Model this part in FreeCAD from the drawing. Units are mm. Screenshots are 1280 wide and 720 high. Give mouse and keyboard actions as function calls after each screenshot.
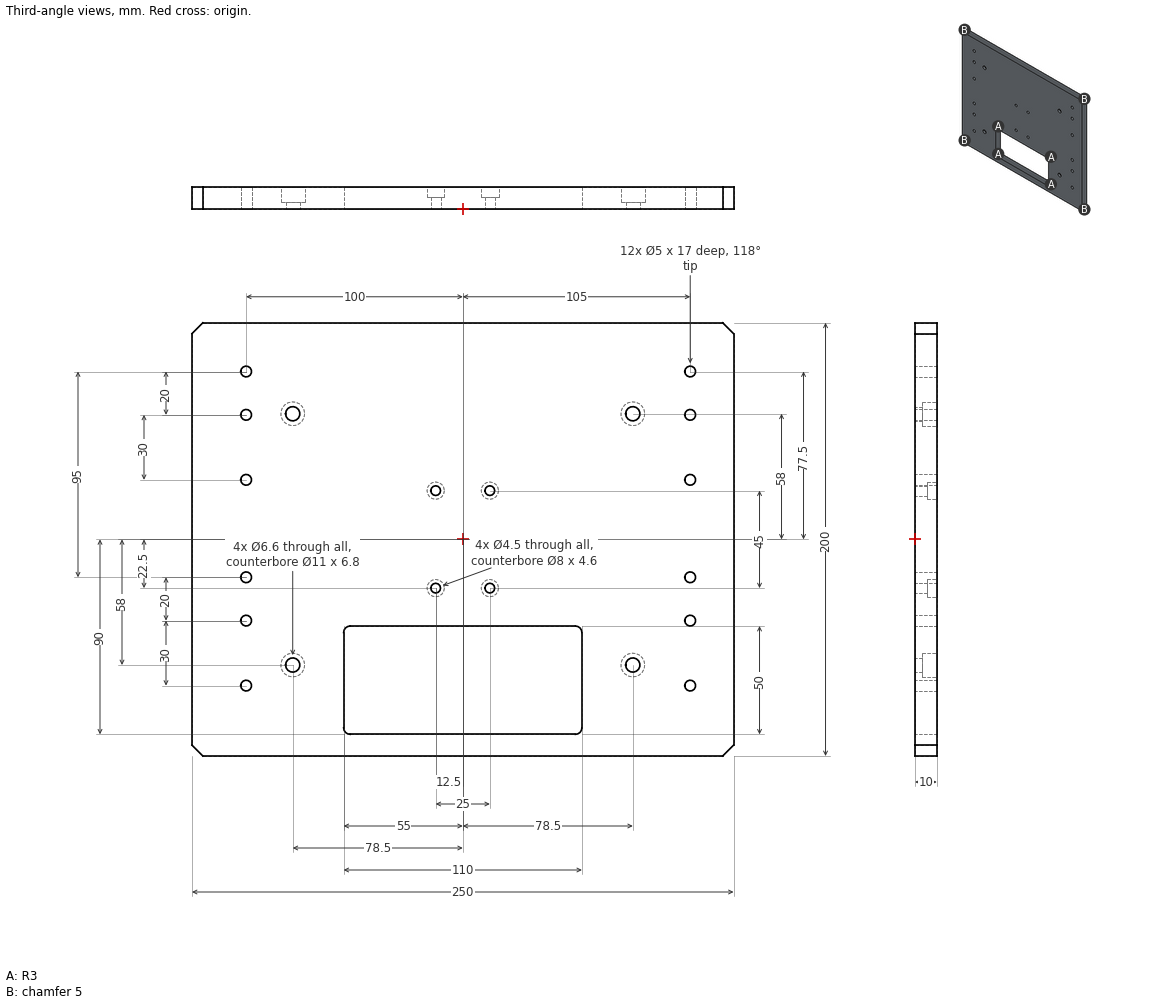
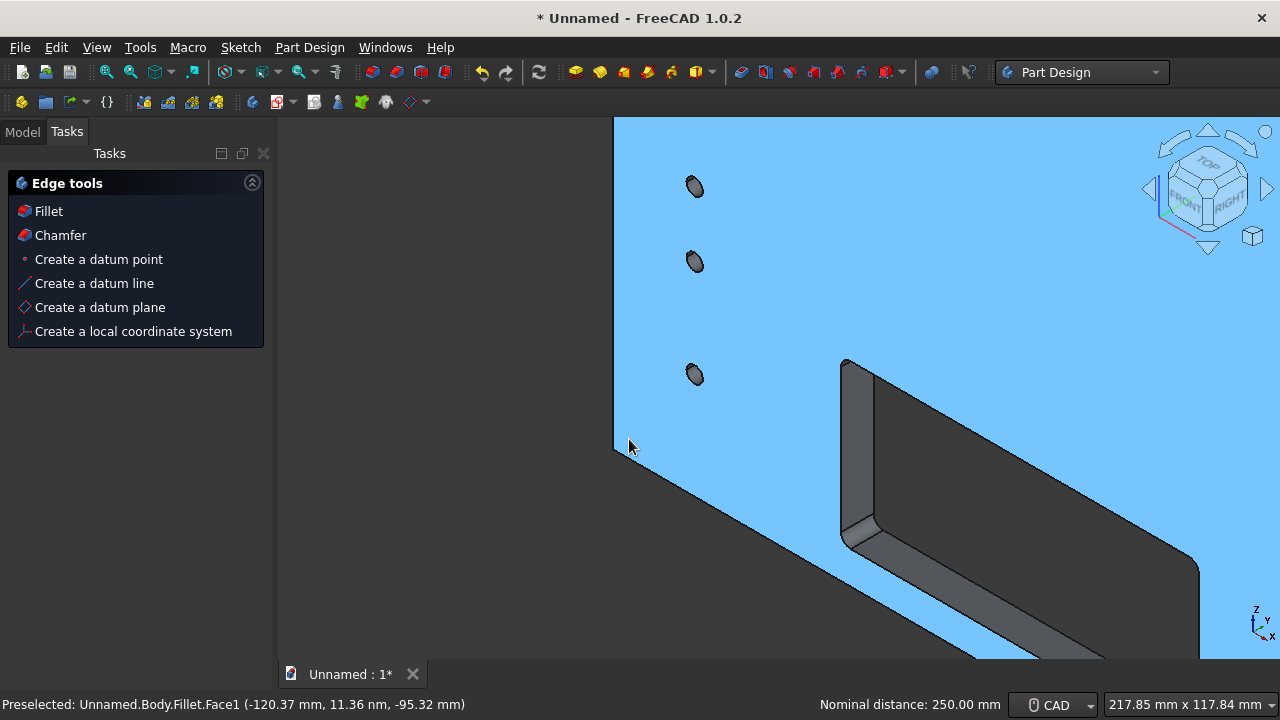
click(108, 72)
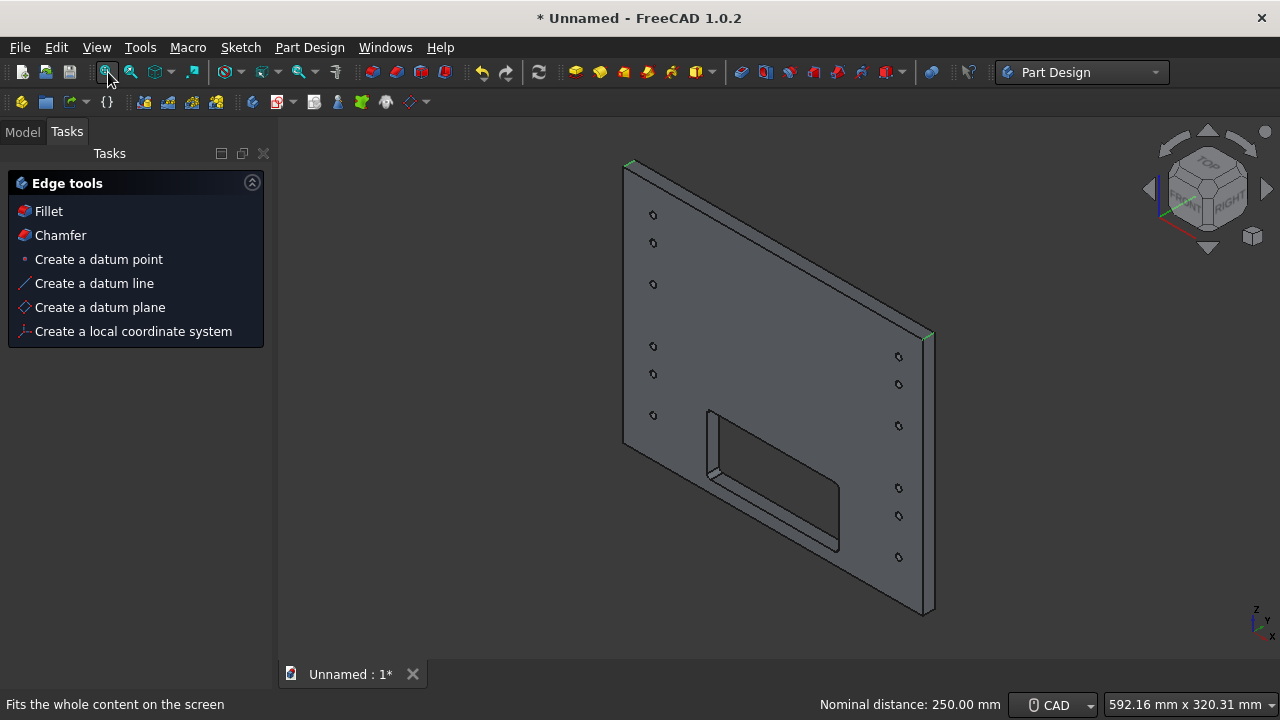
key(1)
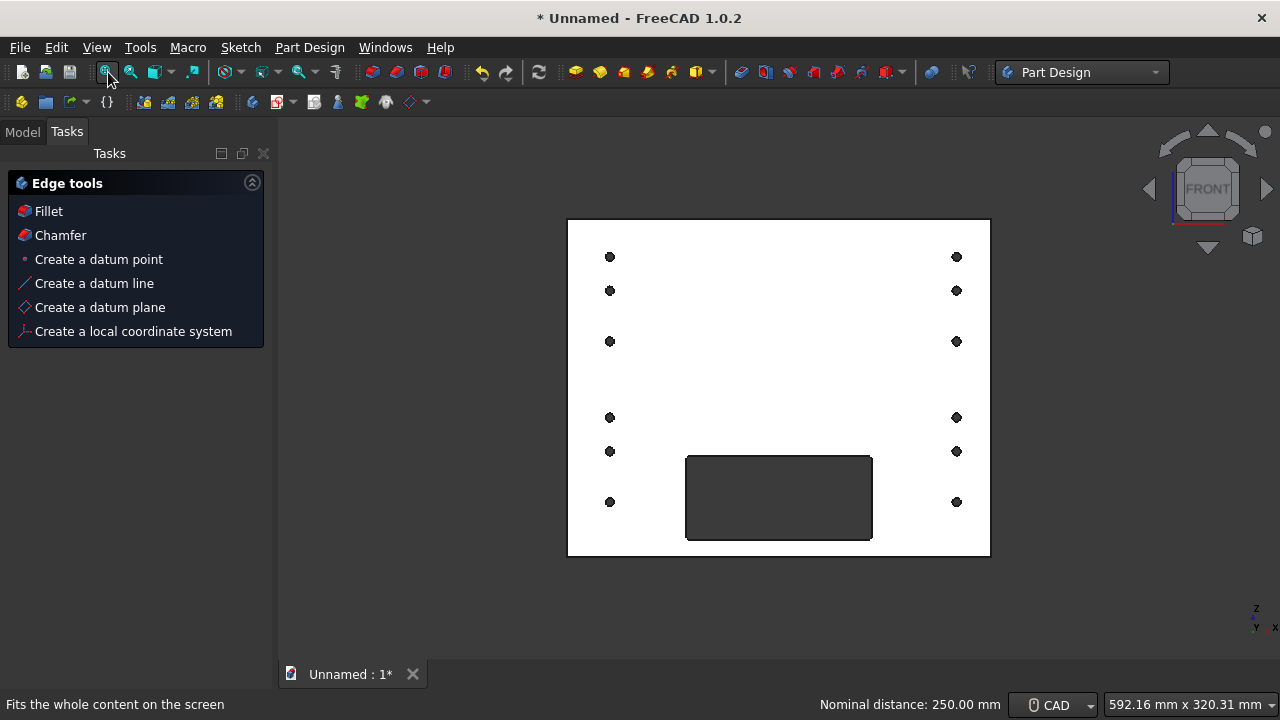
scroll(567, 556, up, 5)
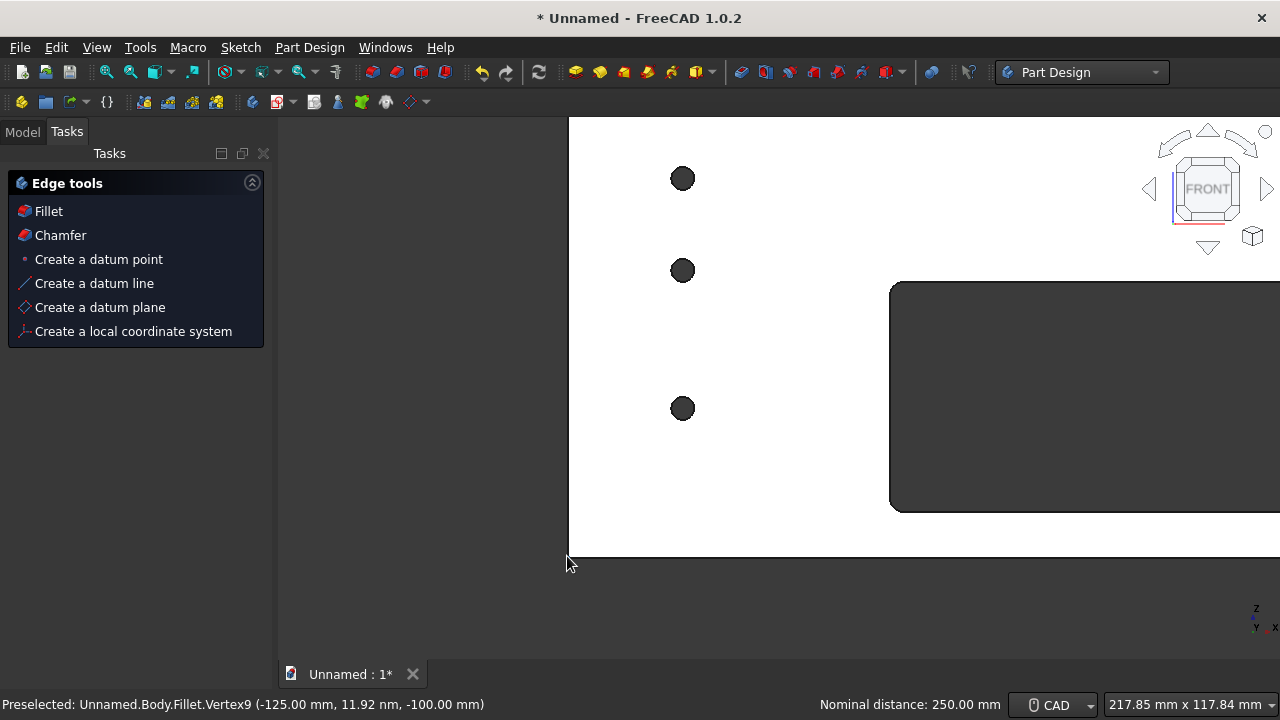
click(108, 72)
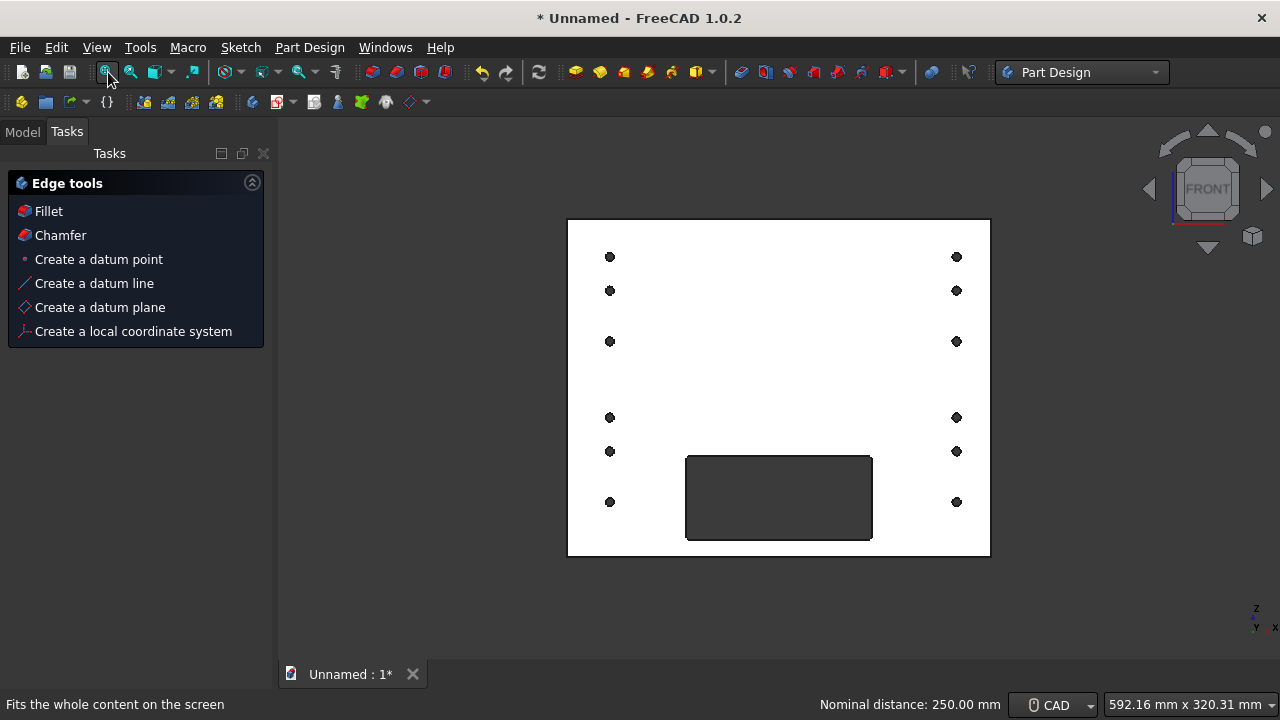
key(3)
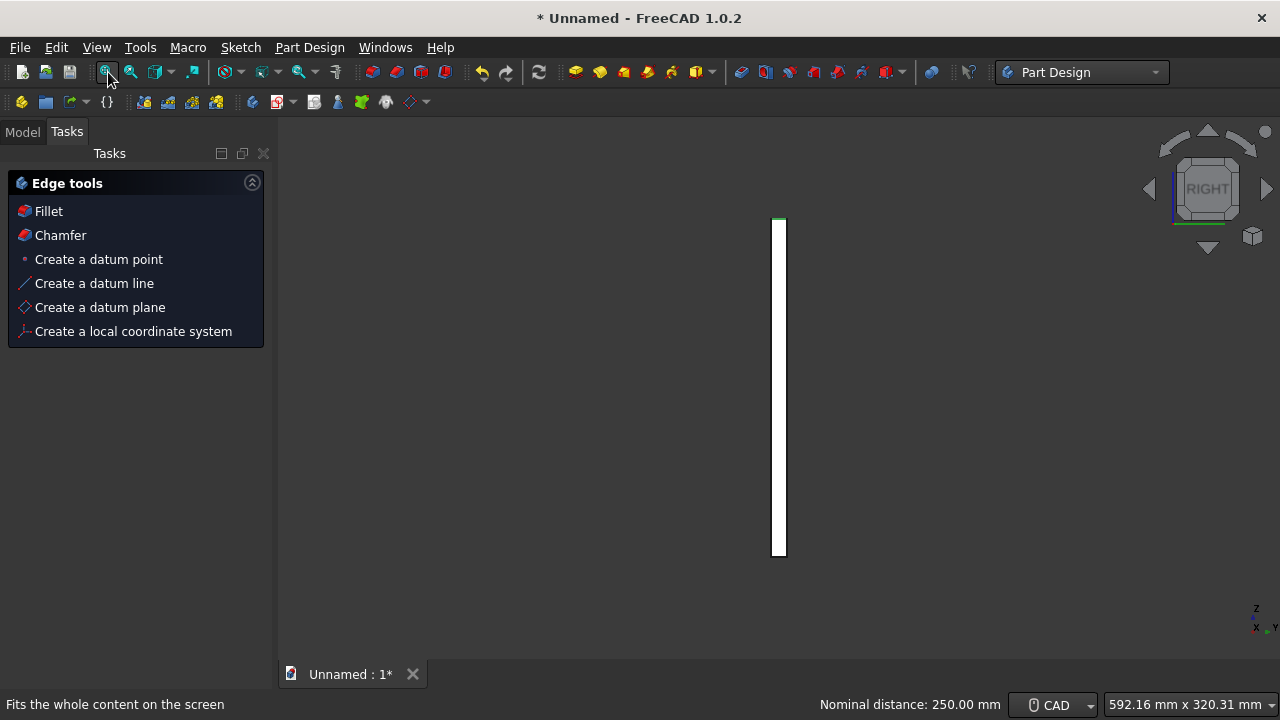
click(779, 556, ctrl)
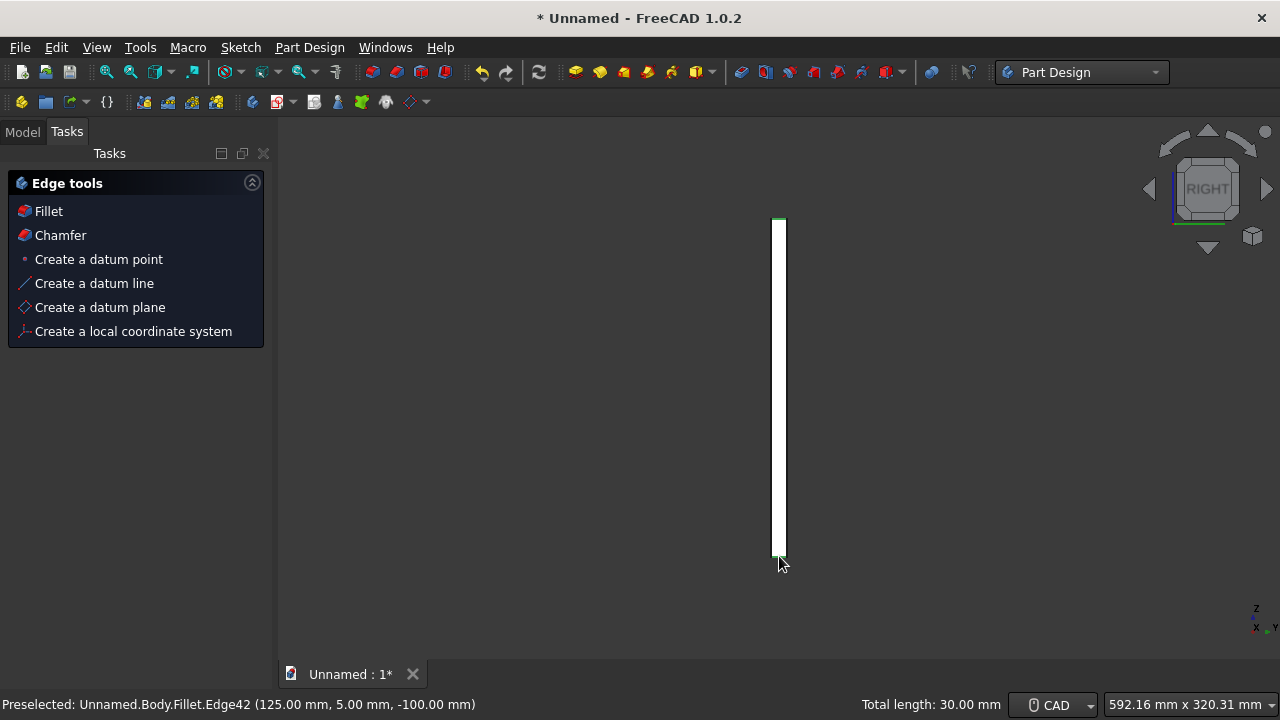
scroll(779, 556, up, 5)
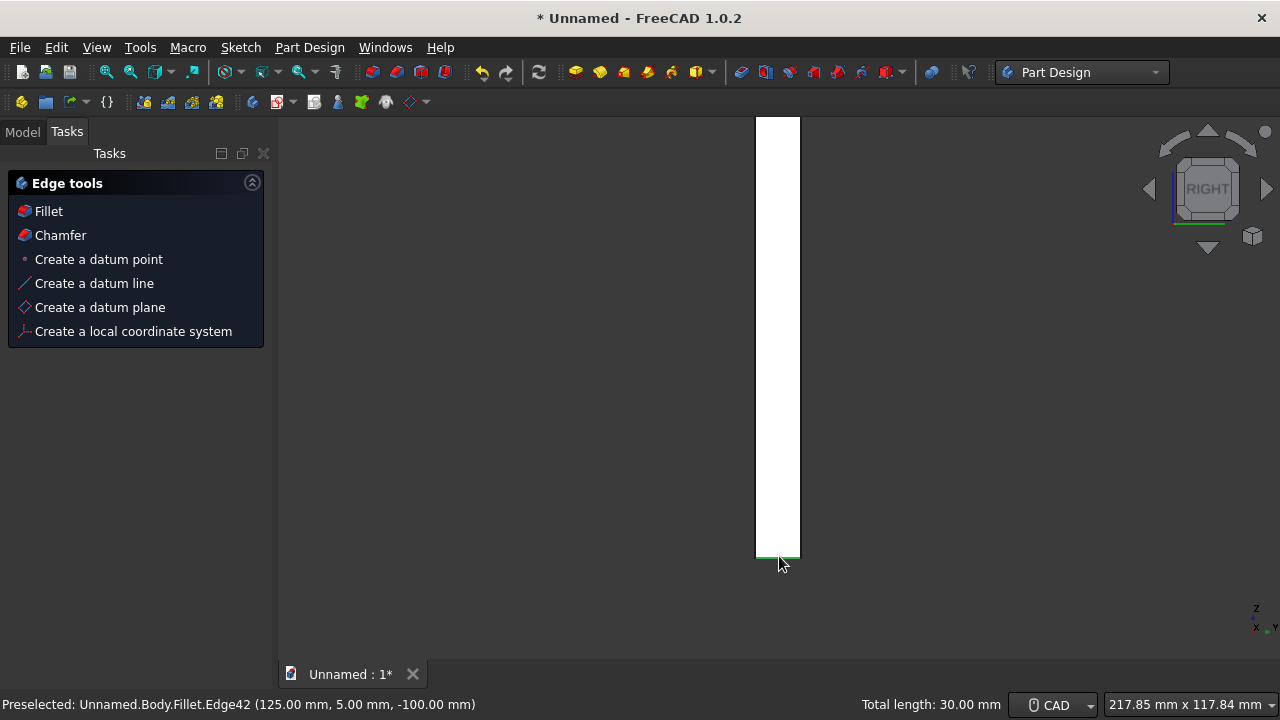
click(108, 72)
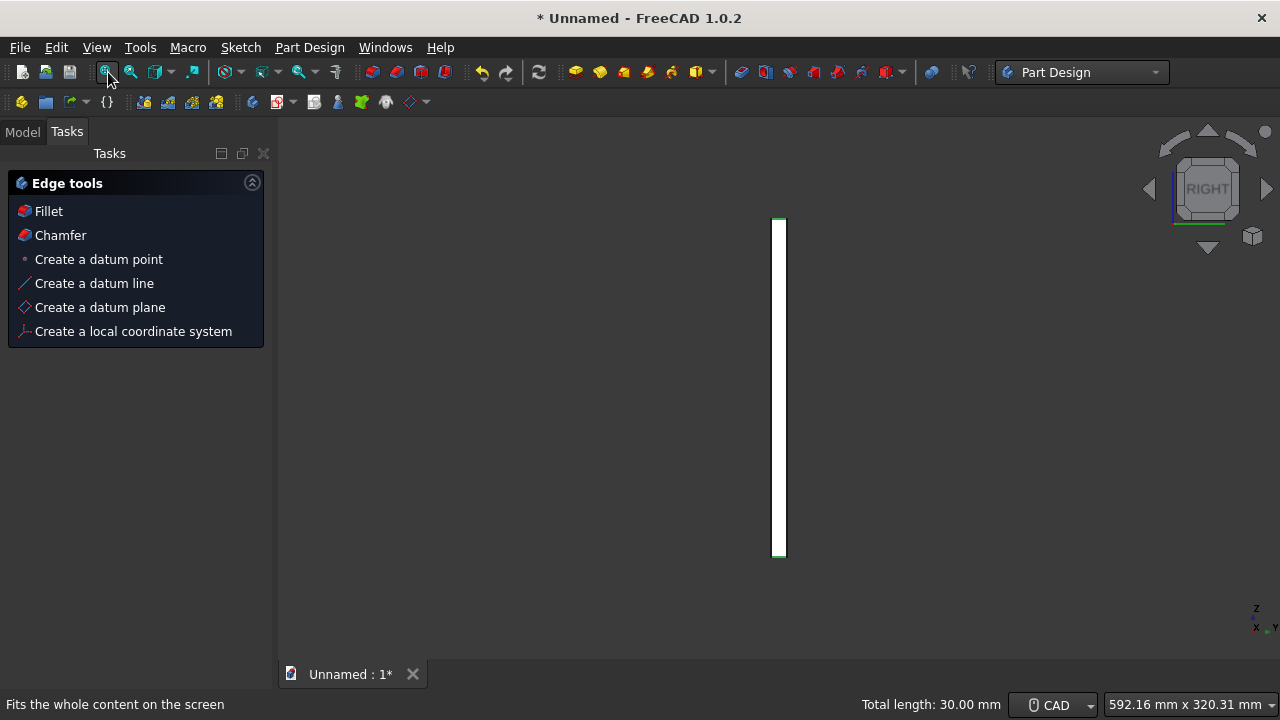
key(5)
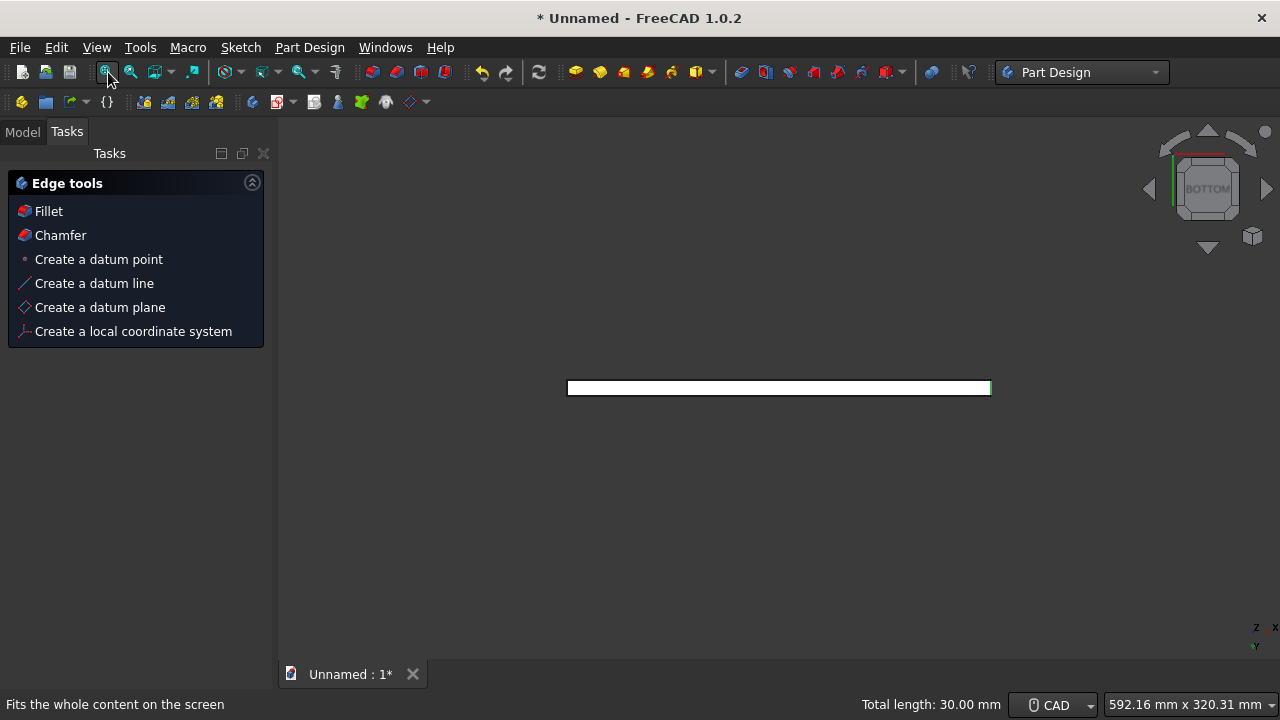
click(108, 72)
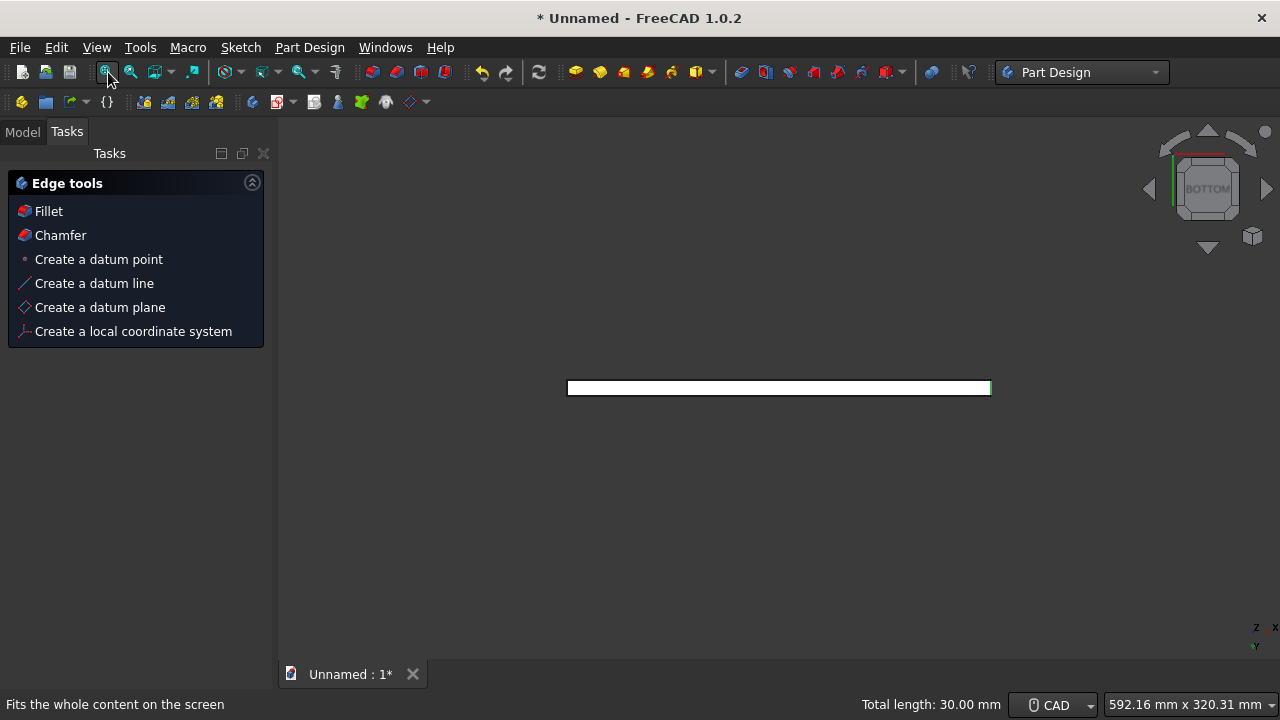
click(567, 387, ctrl)